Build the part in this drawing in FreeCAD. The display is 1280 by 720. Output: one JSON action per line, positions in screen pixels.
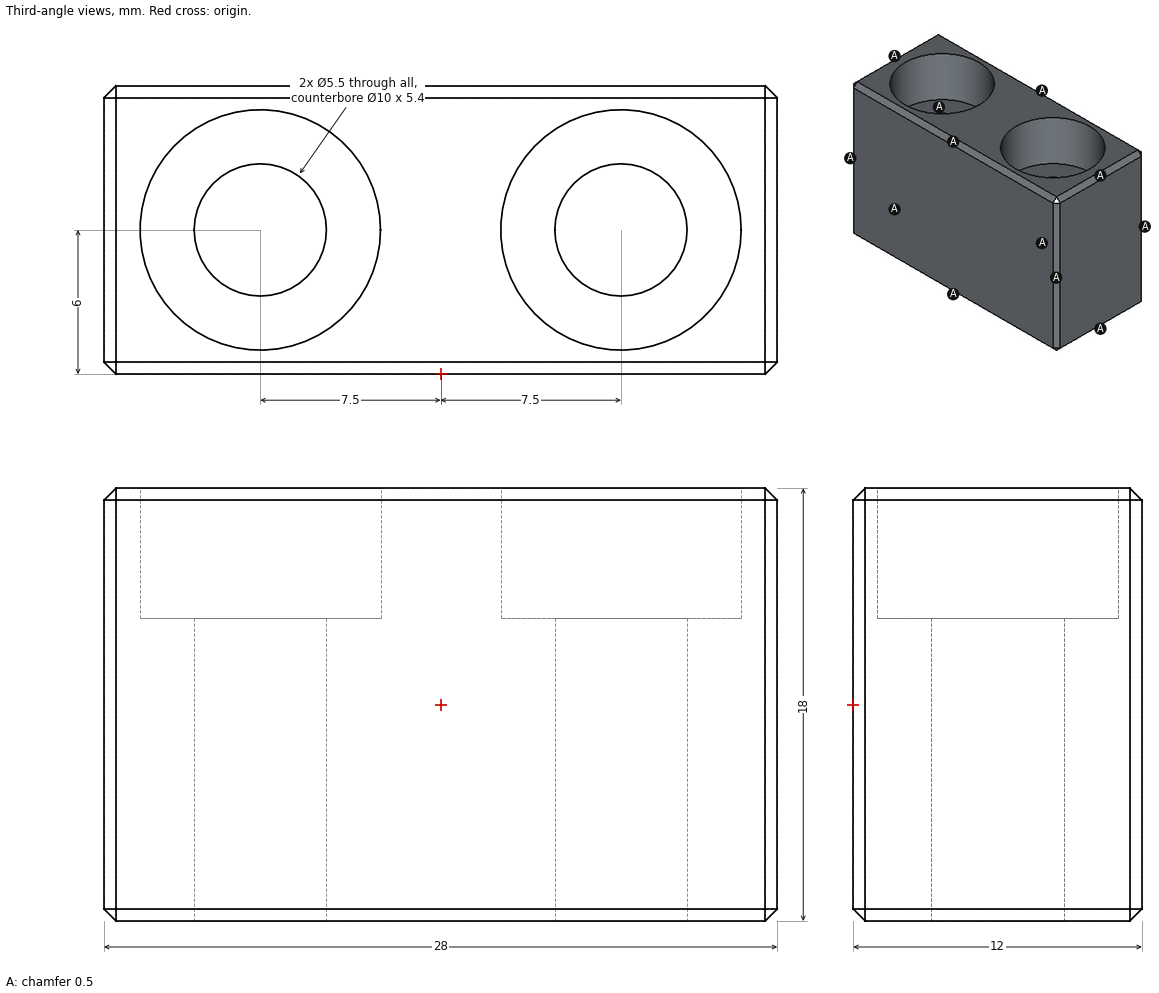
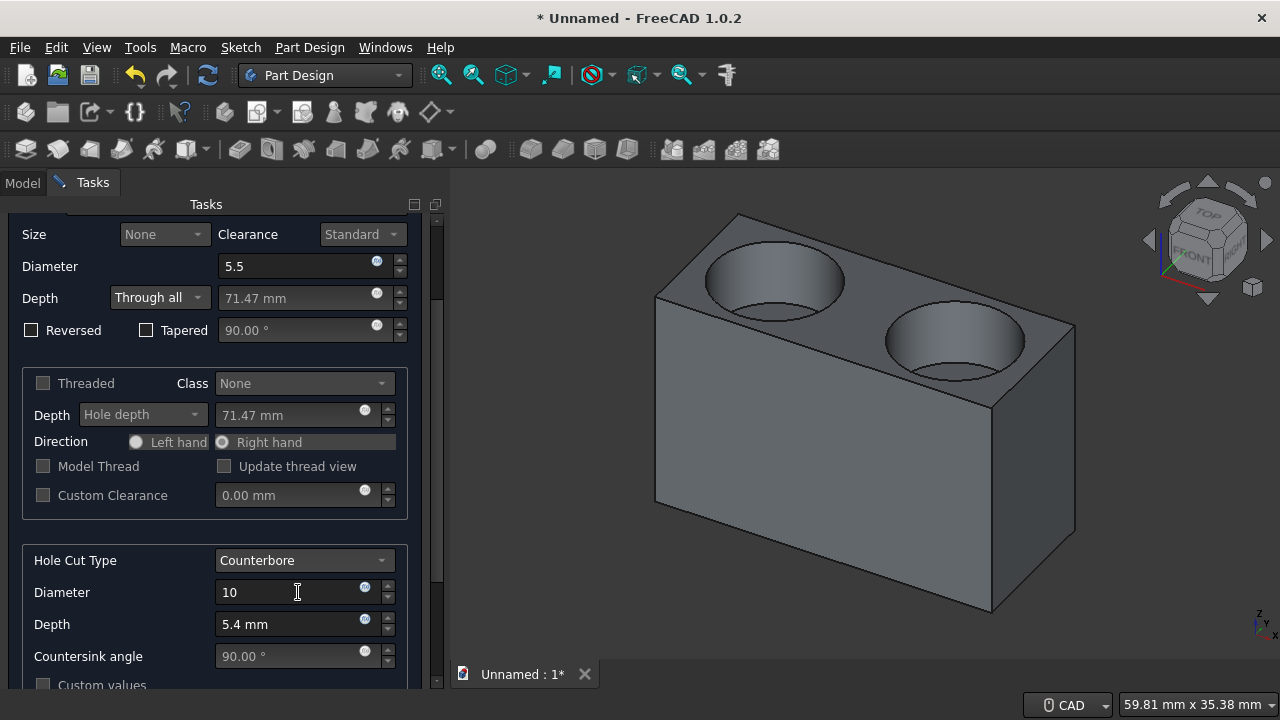
{"action": "scroll", "coordinate": [437, 451], "scroll_direction": "up", "scroll_amount": 3}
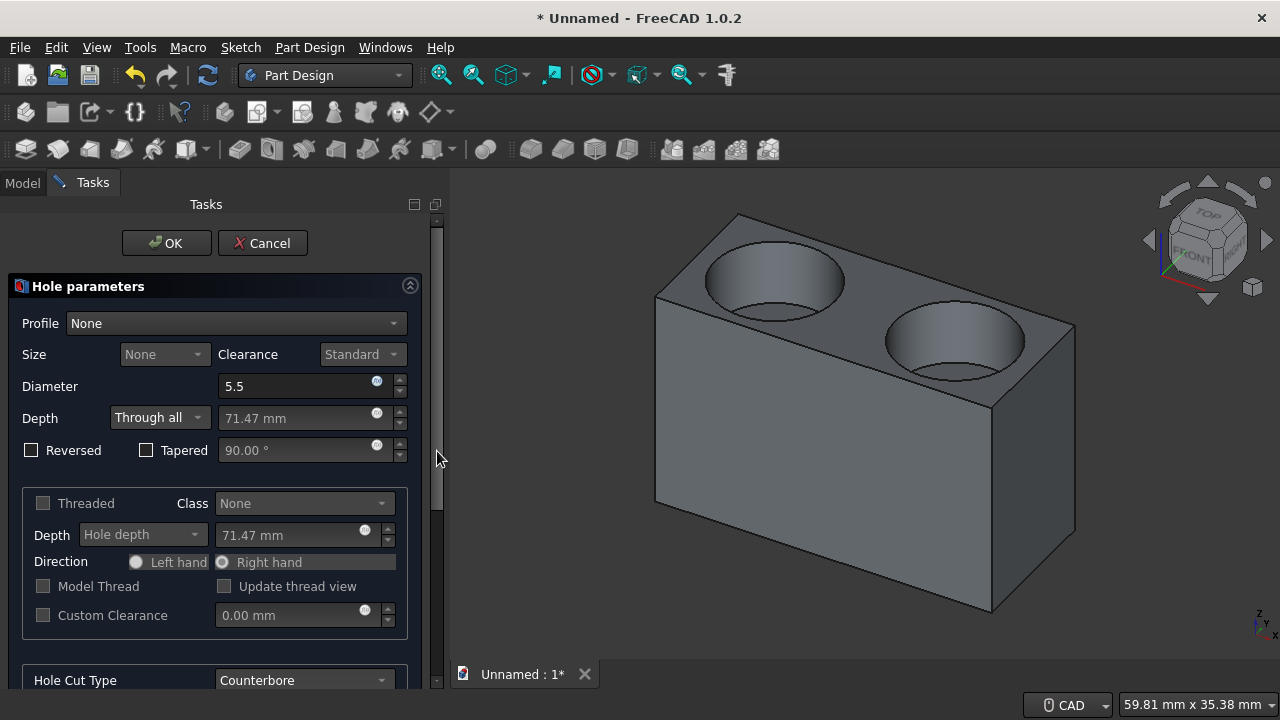
{"action": "left_click", "coordinate": [167, 243]}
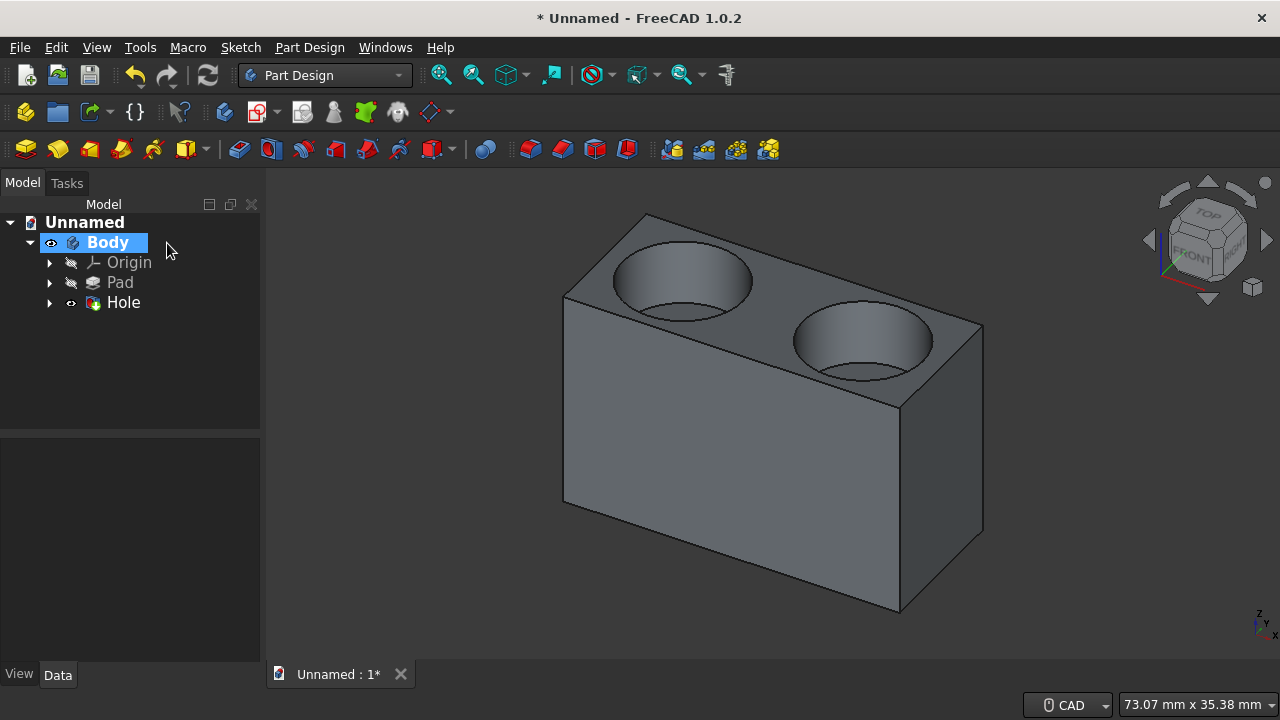
{"action": "left_click", "coordinate": [779, 470]}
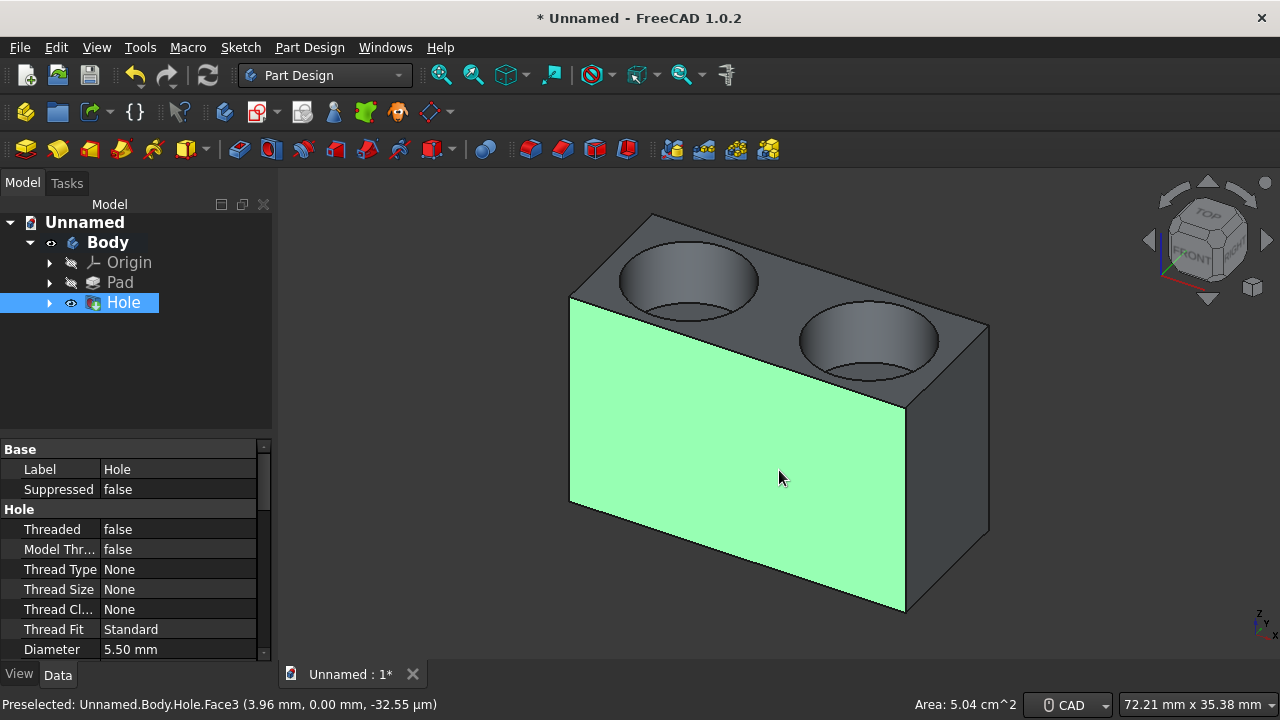
{"action": "left_click", "coordinate": [947, 366], "text": "ctrl"}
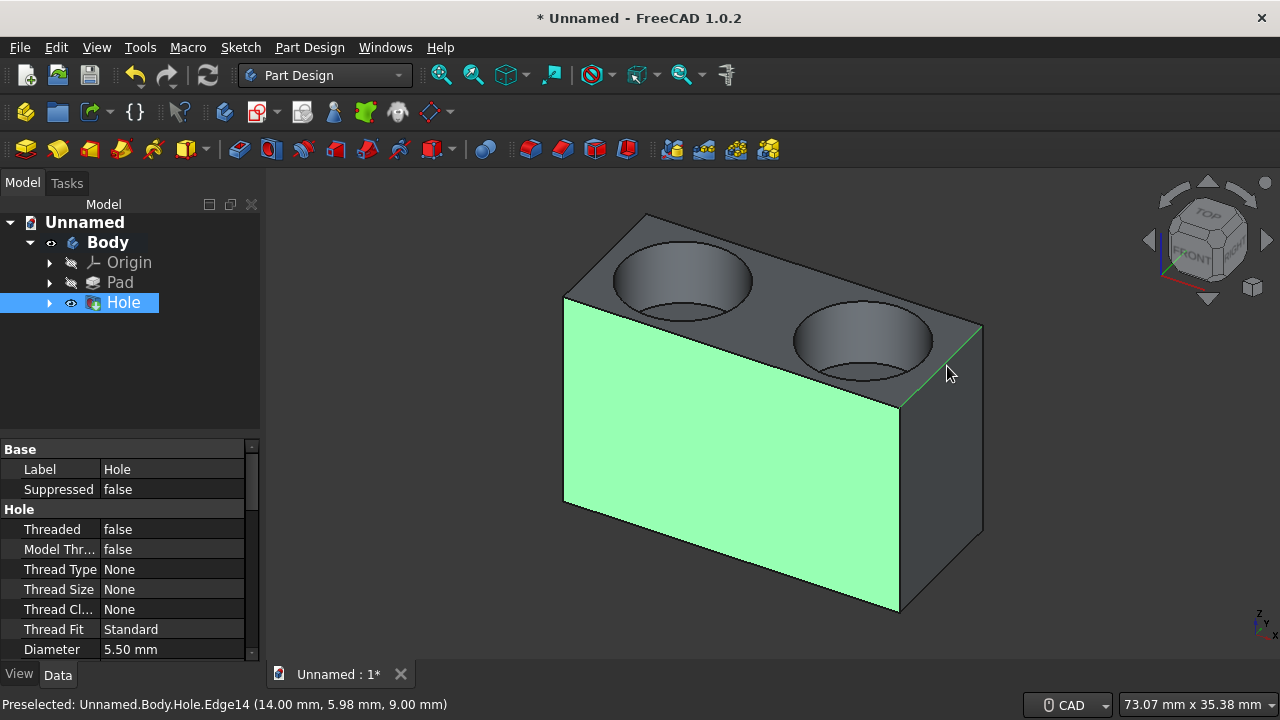
{"action": "key", "text": "0"}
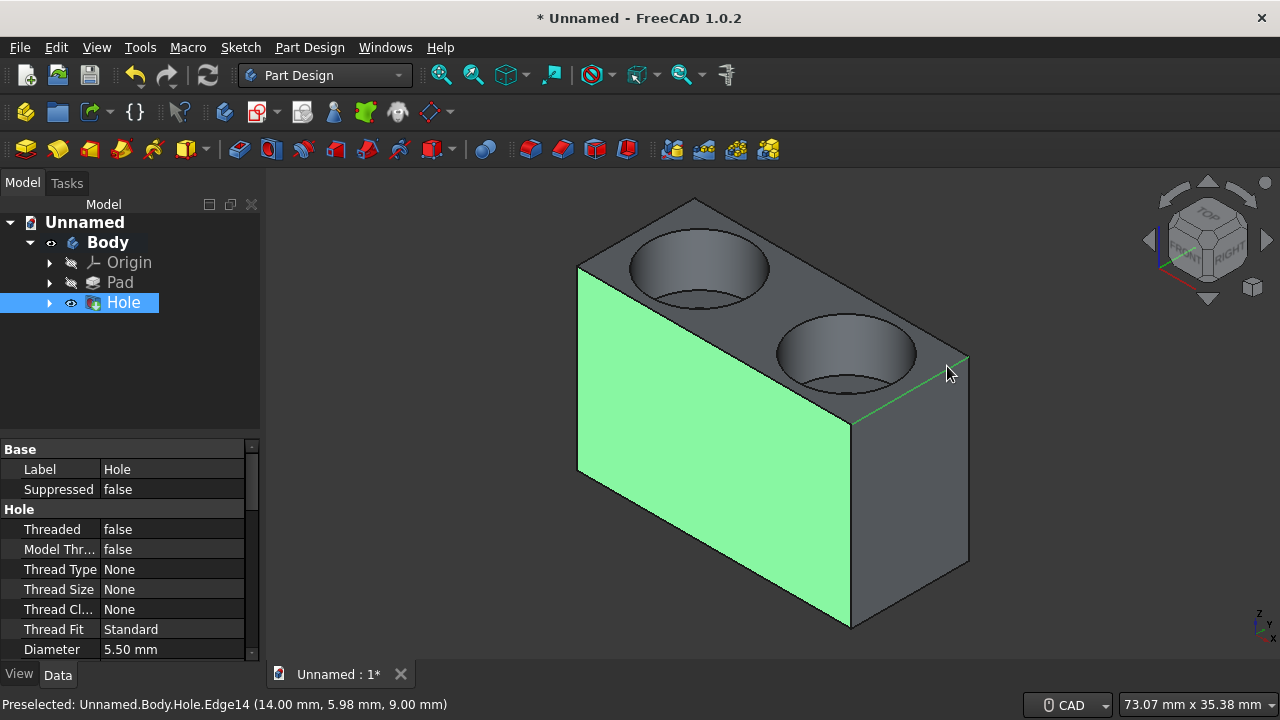
{"action": "key", "text": "2"}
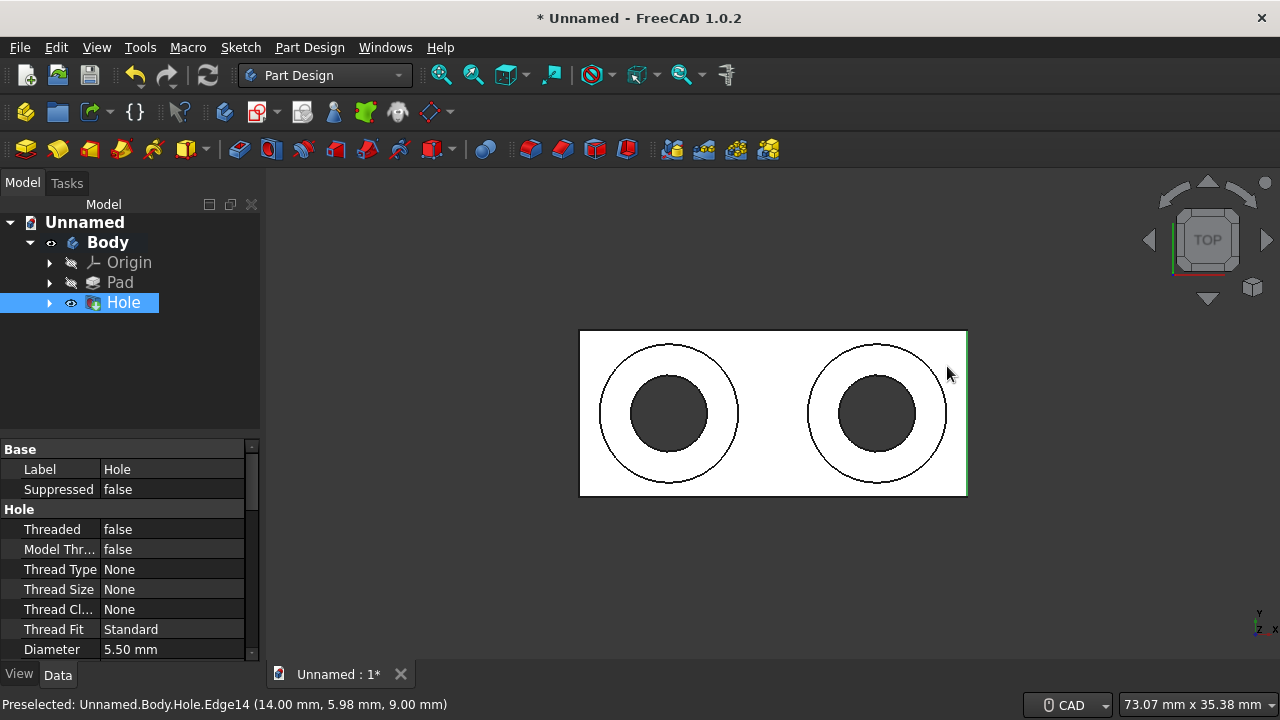
{"action": "left_click", "coordinate": [442, 76]}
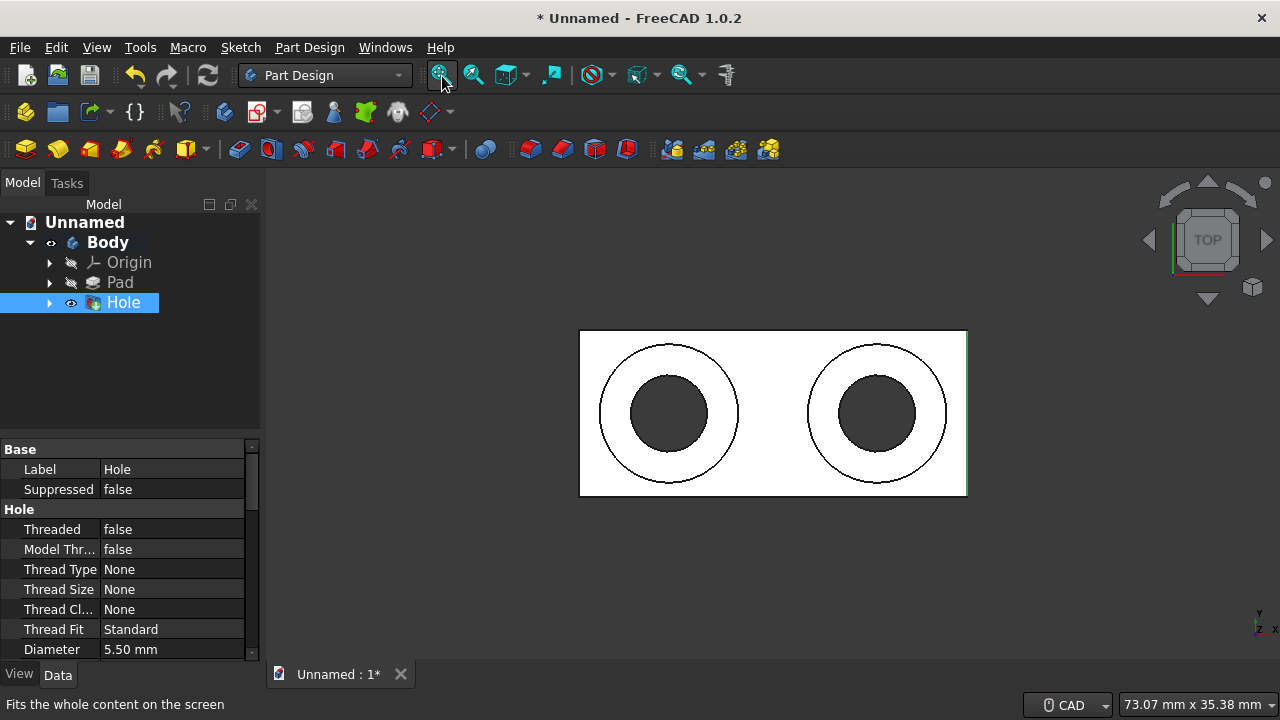
{"action": "left_click", "coordinate": [579, 413], "text": "ctrl"}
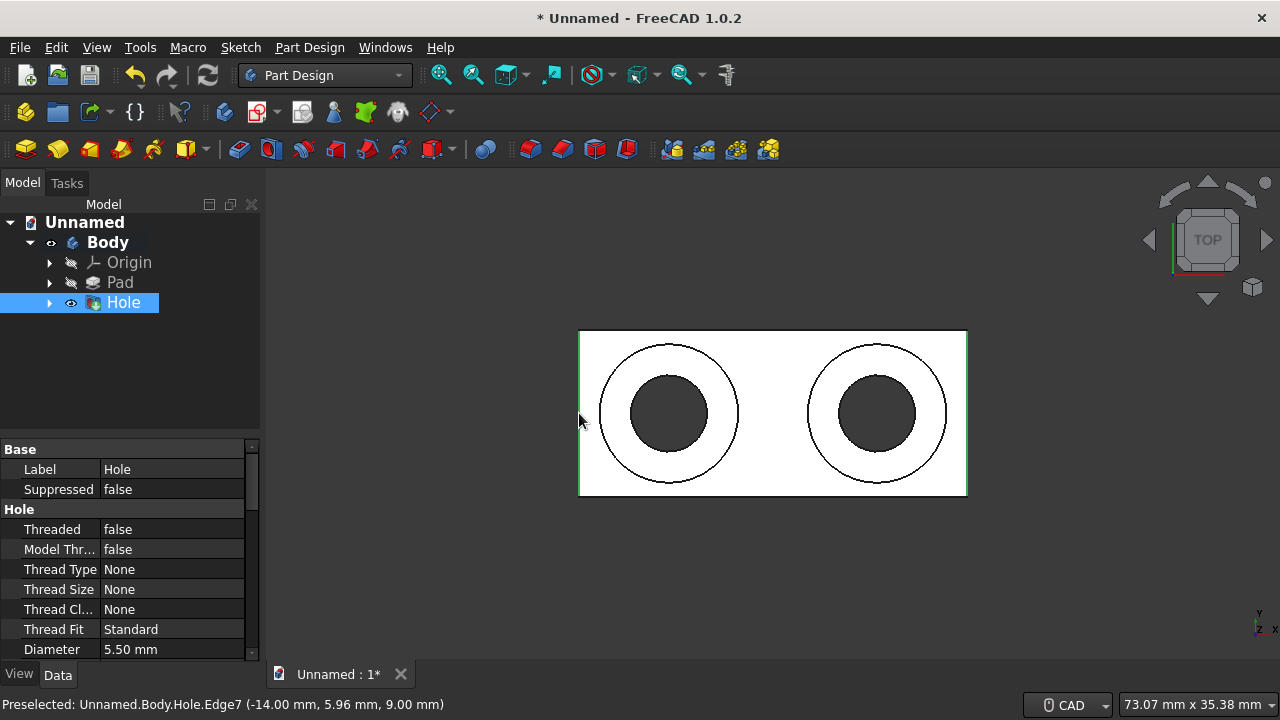
{"action": "key", "text": "1"}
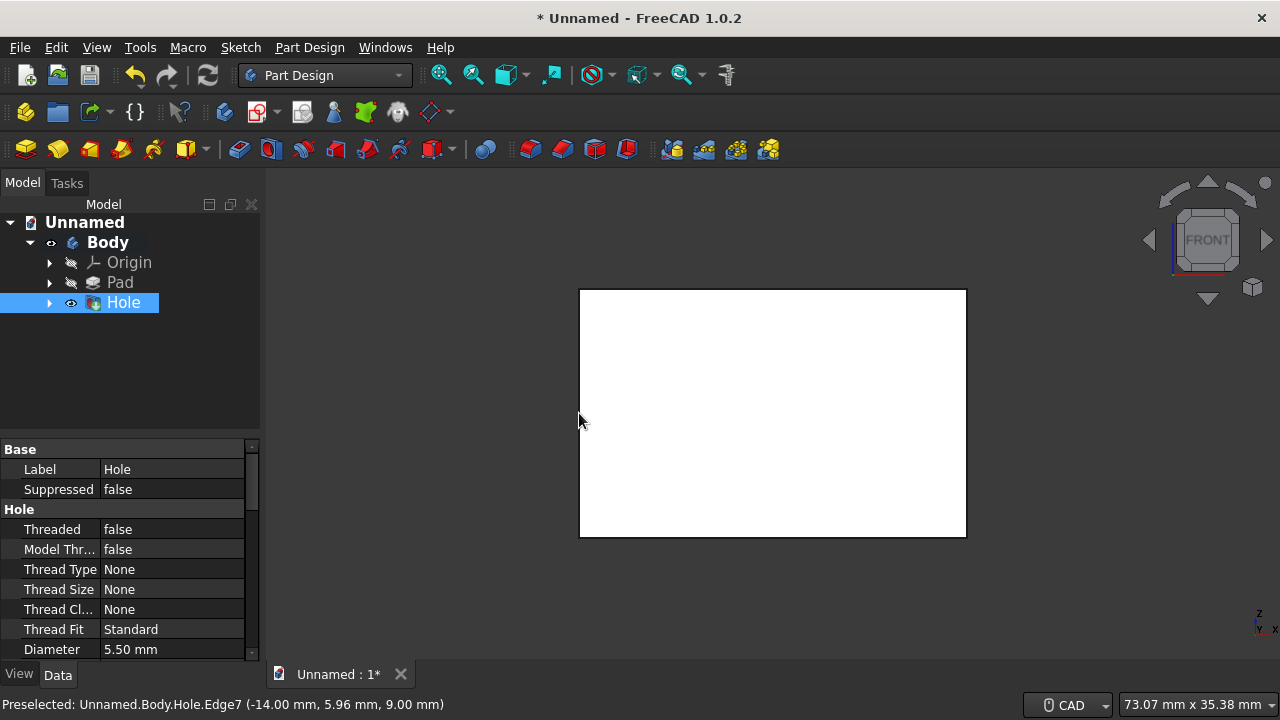
{"action": "key", "text": "3"}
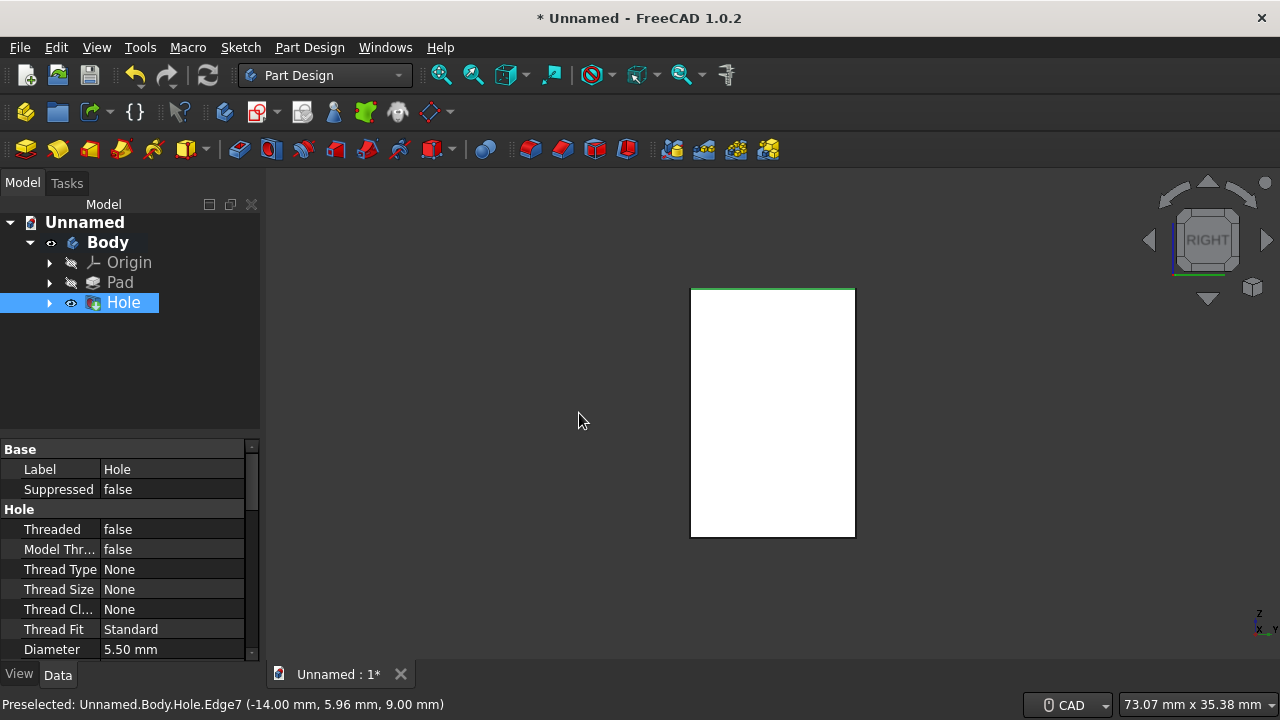
{"action": "left_click", "coordinate": [773, 537], "text": "ctrl"}